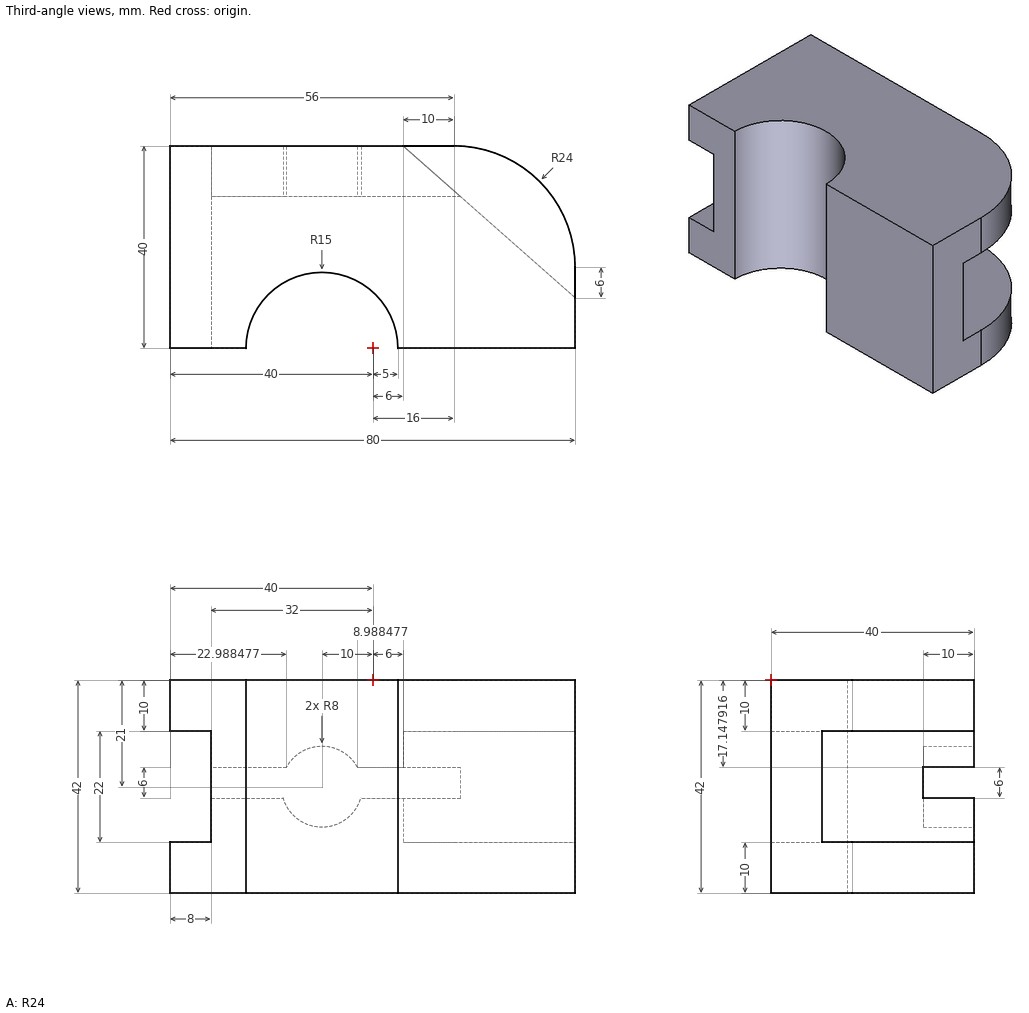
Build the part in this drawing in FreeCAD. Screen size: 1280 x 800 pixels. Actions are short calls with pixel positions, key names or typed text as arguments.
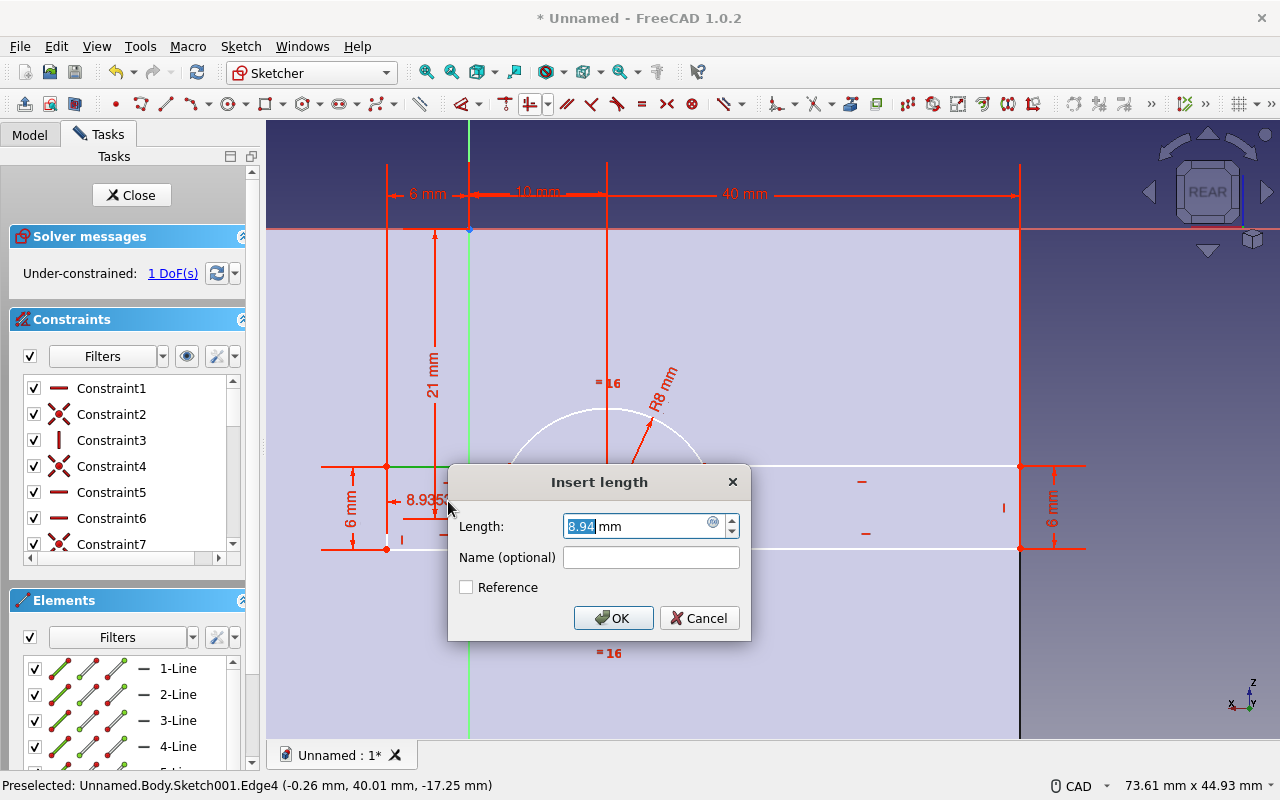
text(8.988477)
key(Return)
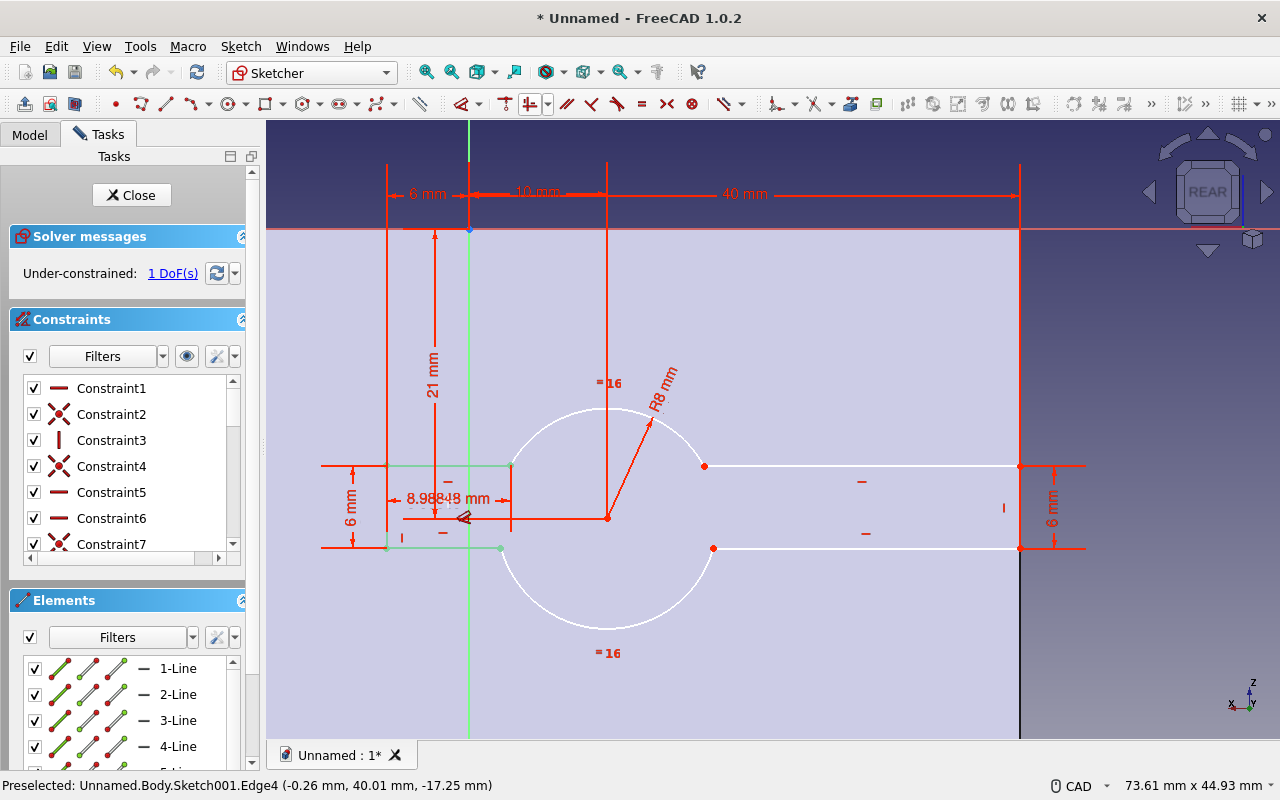
click(926, 466)
click(862, 500)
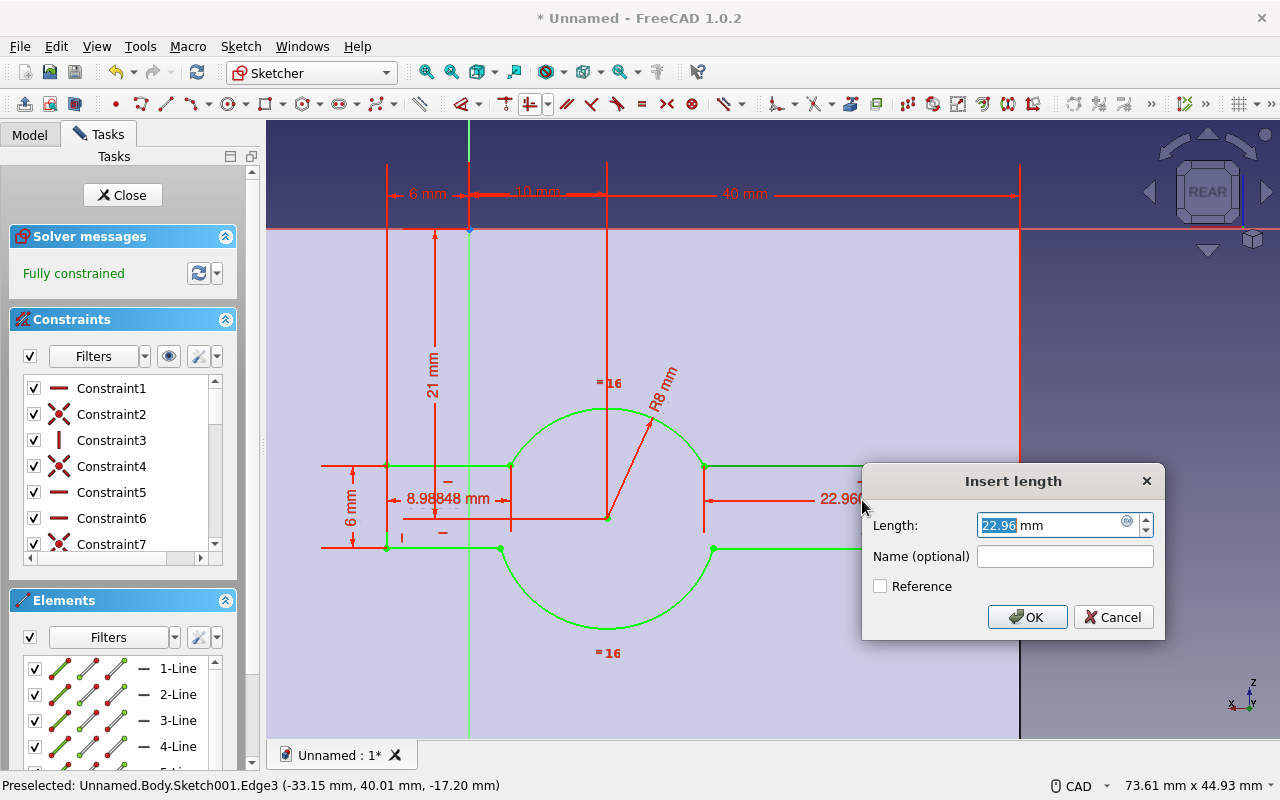
text(22.988477)
key(Return)
key(Escape)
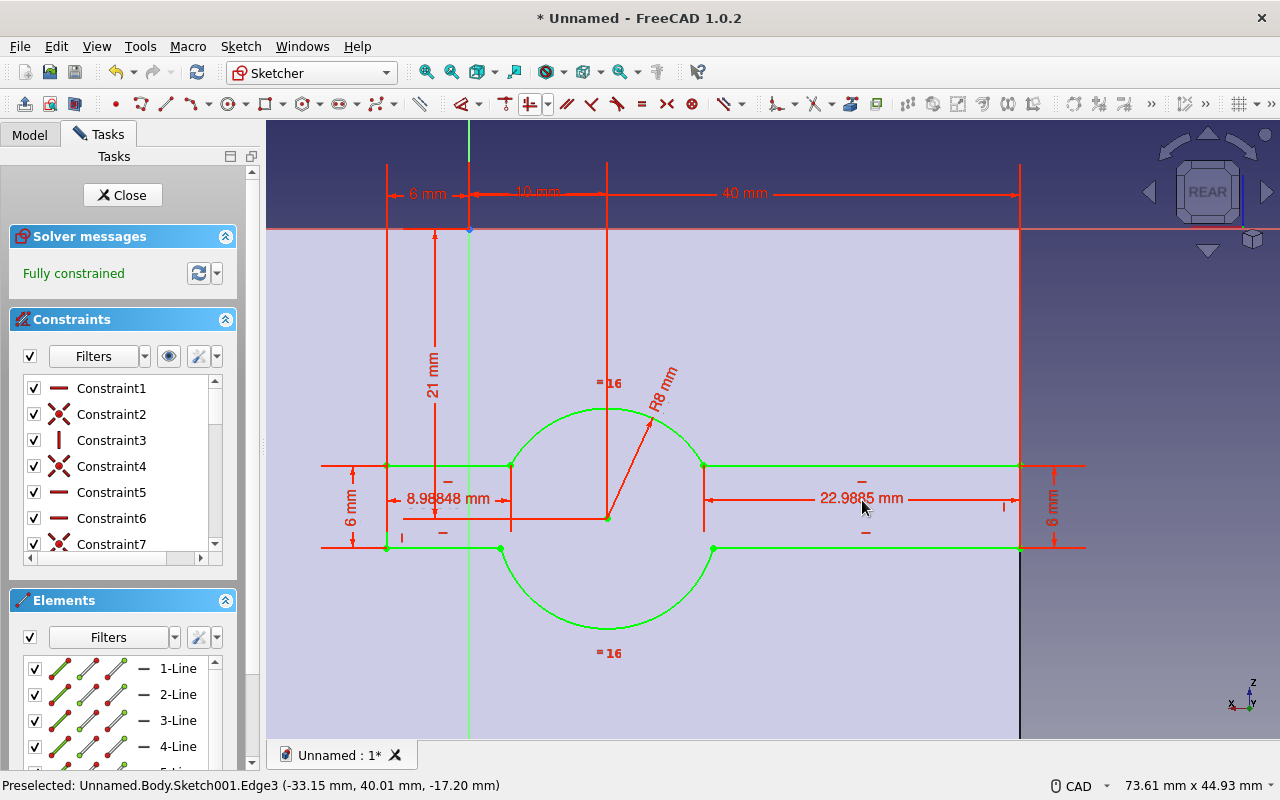
click(123, 195)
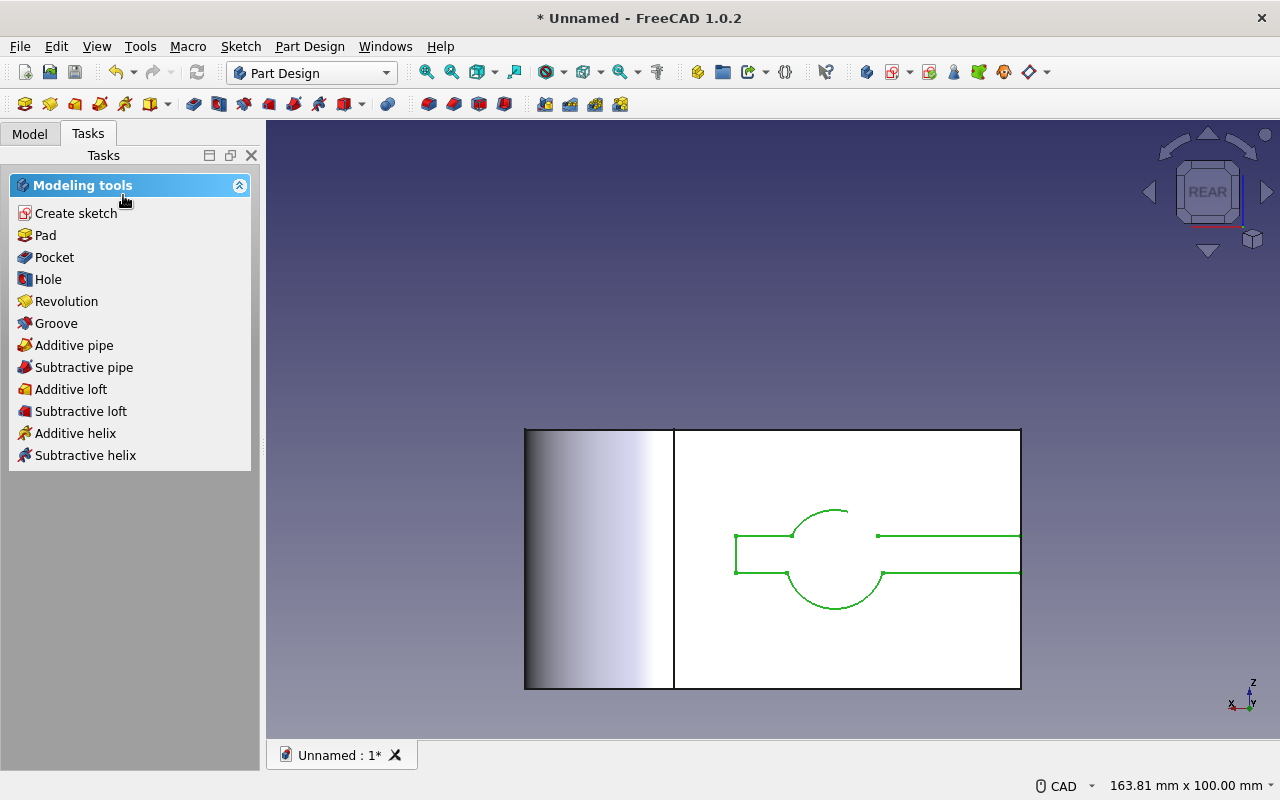
click(194, 104)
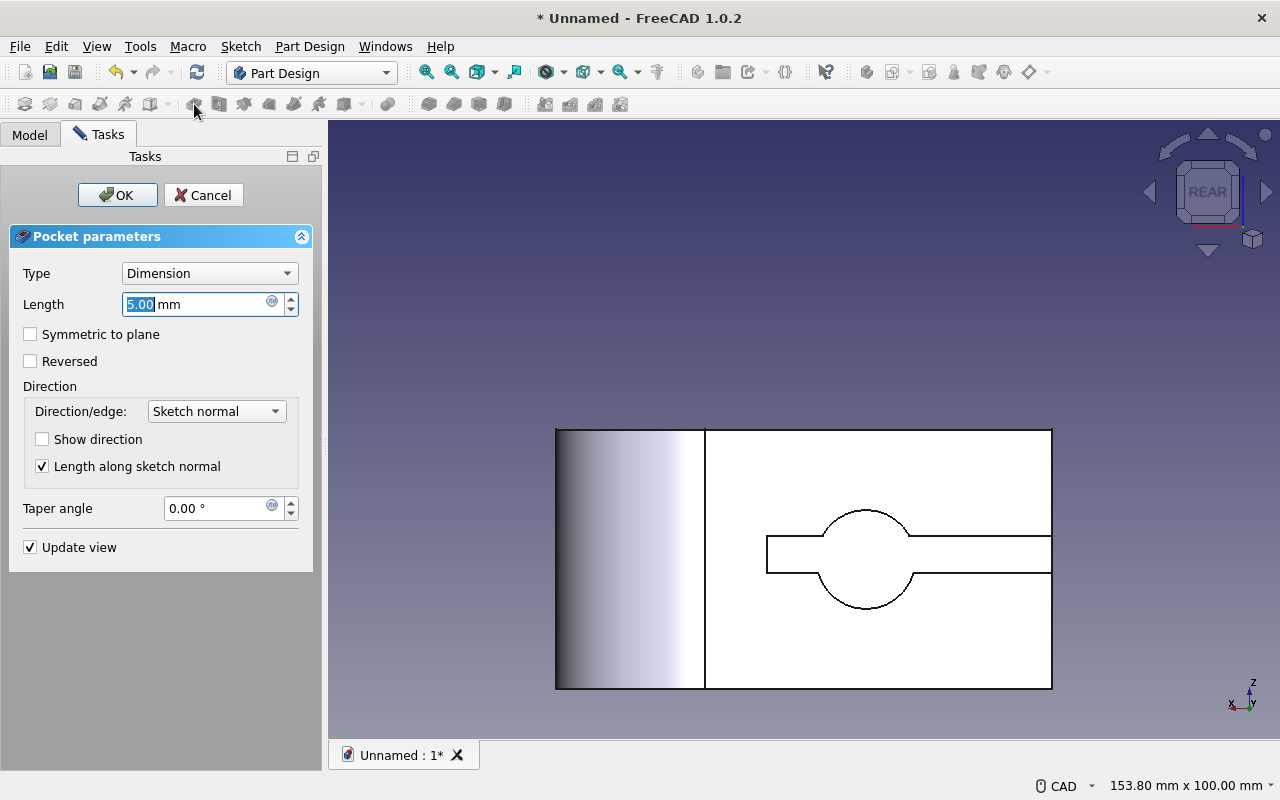
text(10)
key(Tab)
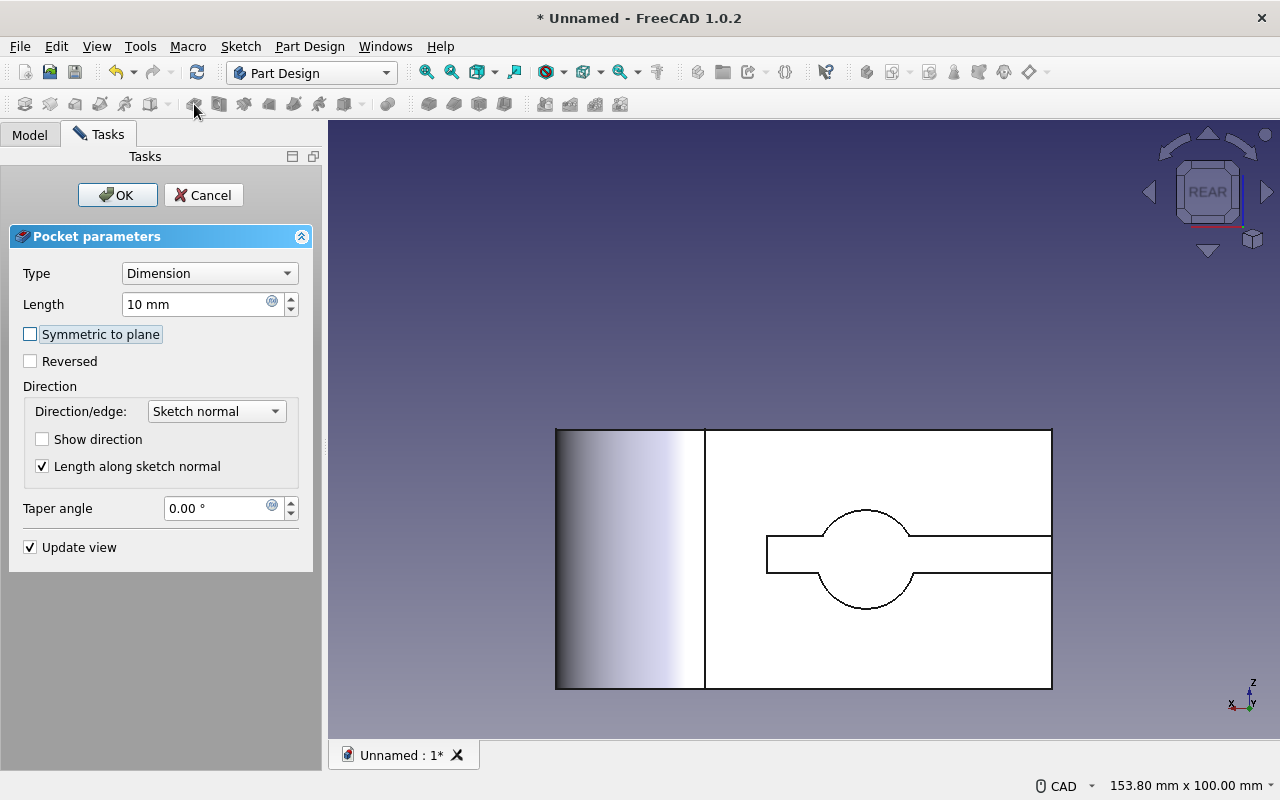
click(118, 195)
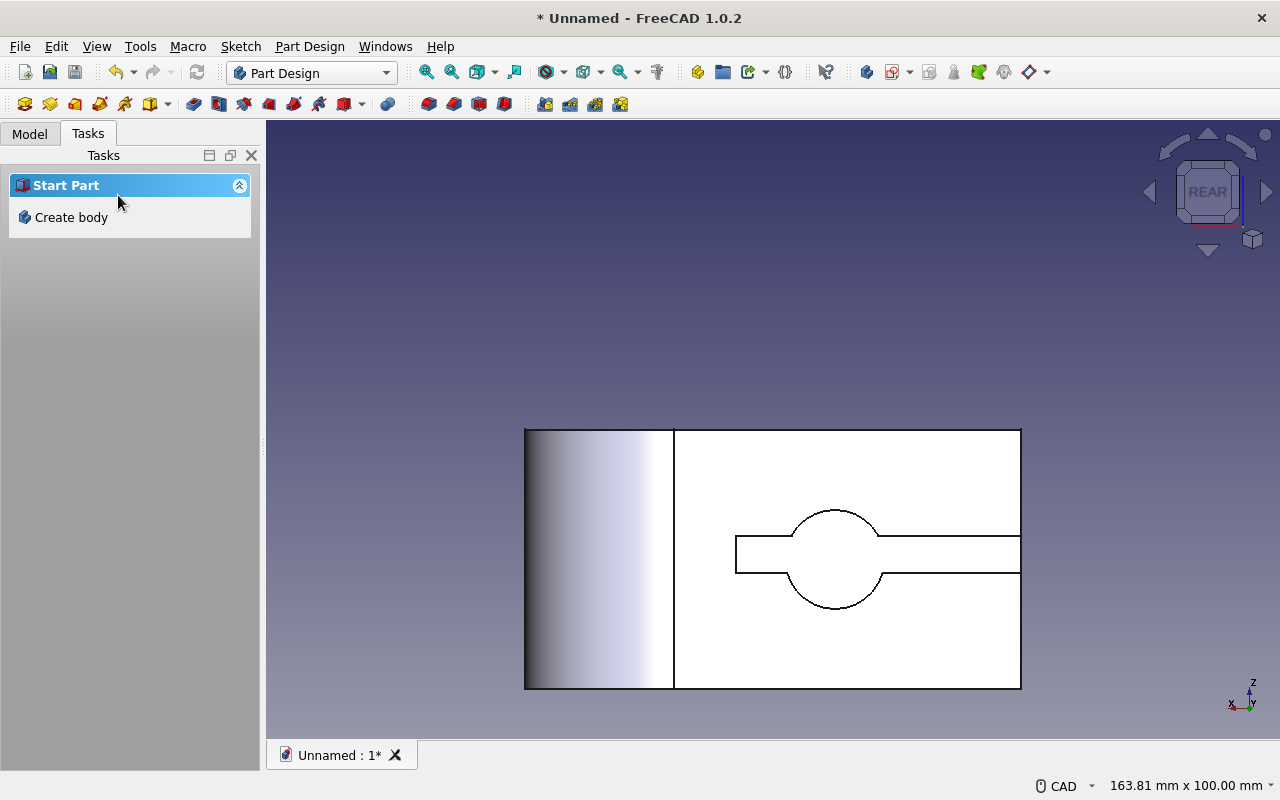
key(0)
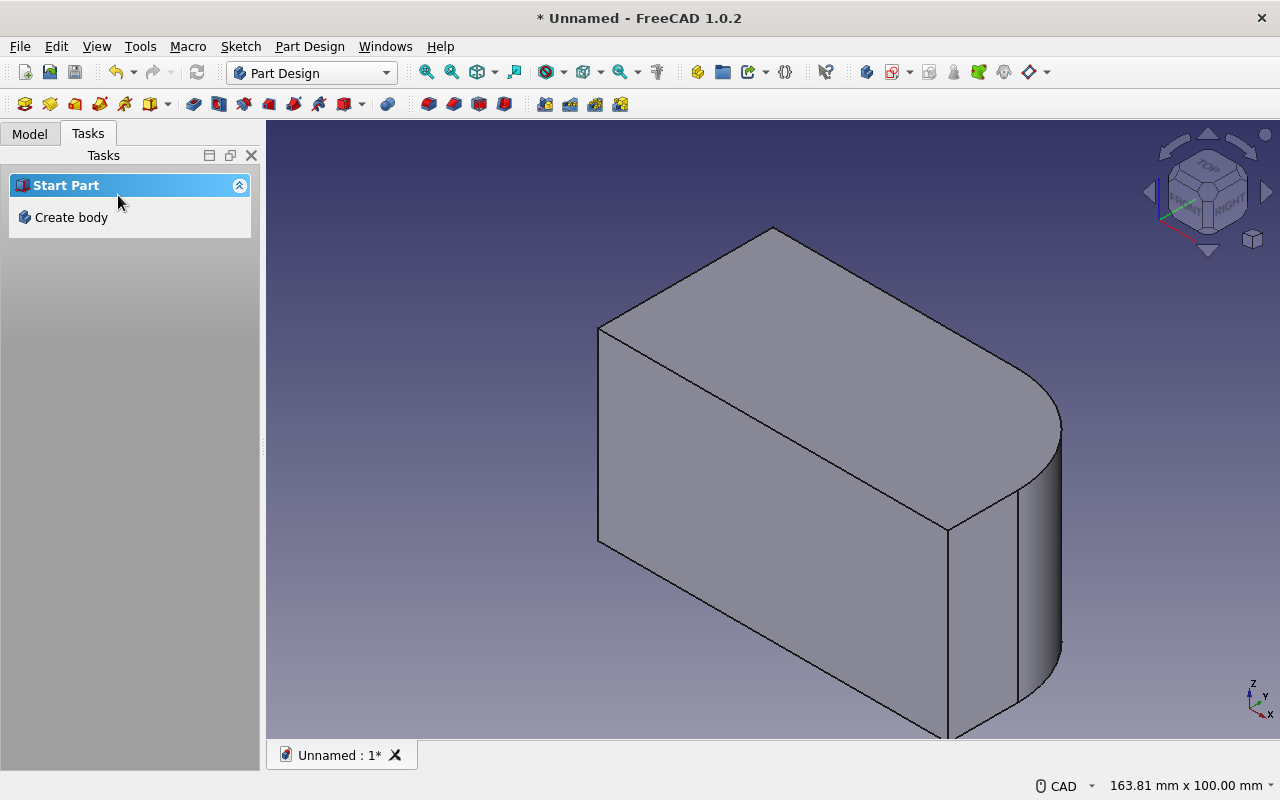
key(v)
key(f)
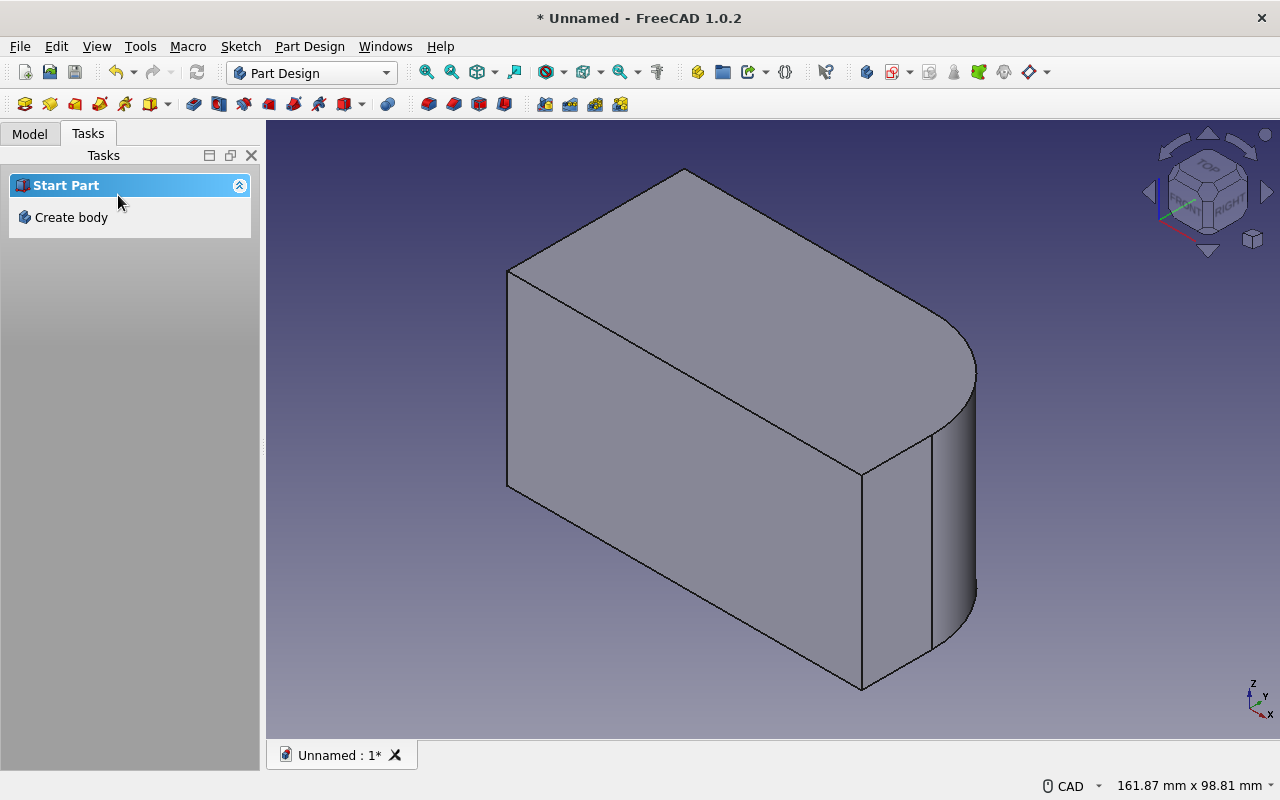
click(824, 350)